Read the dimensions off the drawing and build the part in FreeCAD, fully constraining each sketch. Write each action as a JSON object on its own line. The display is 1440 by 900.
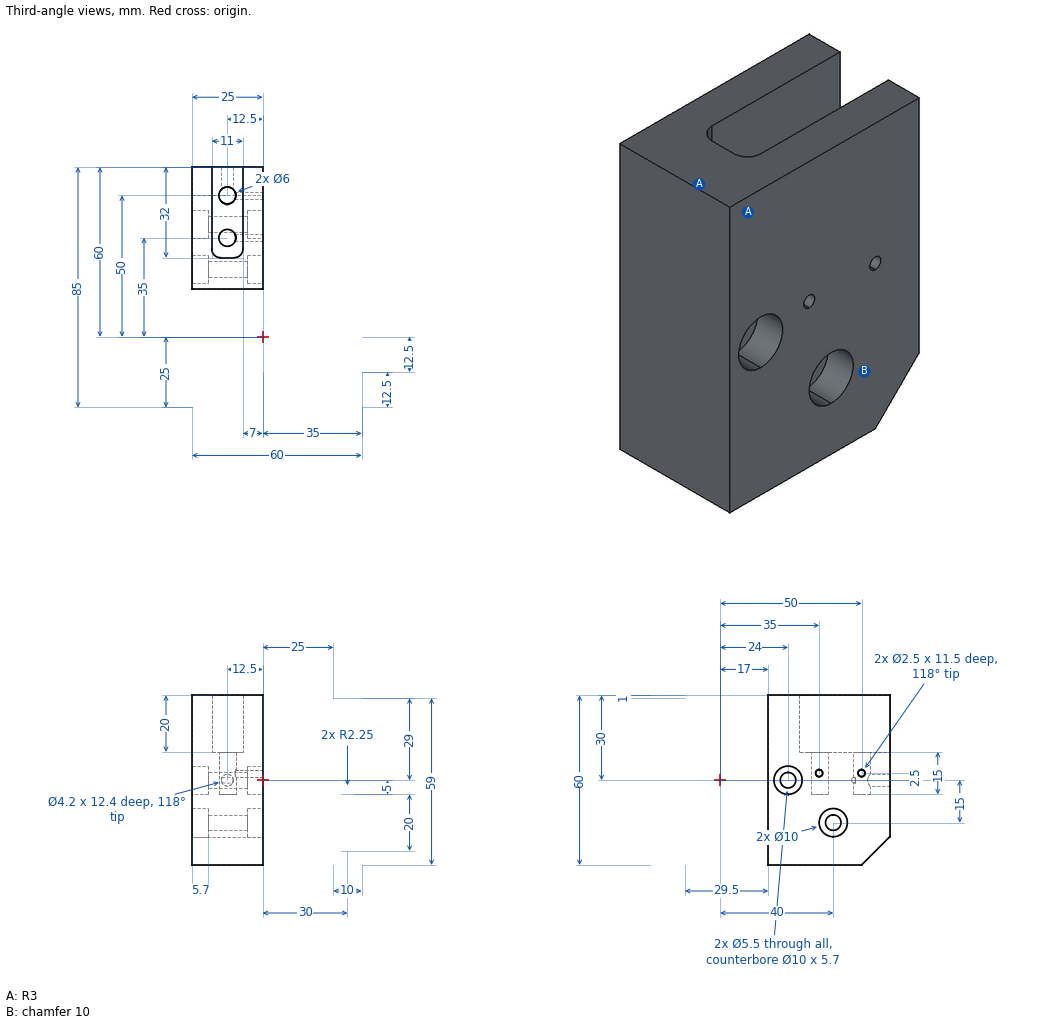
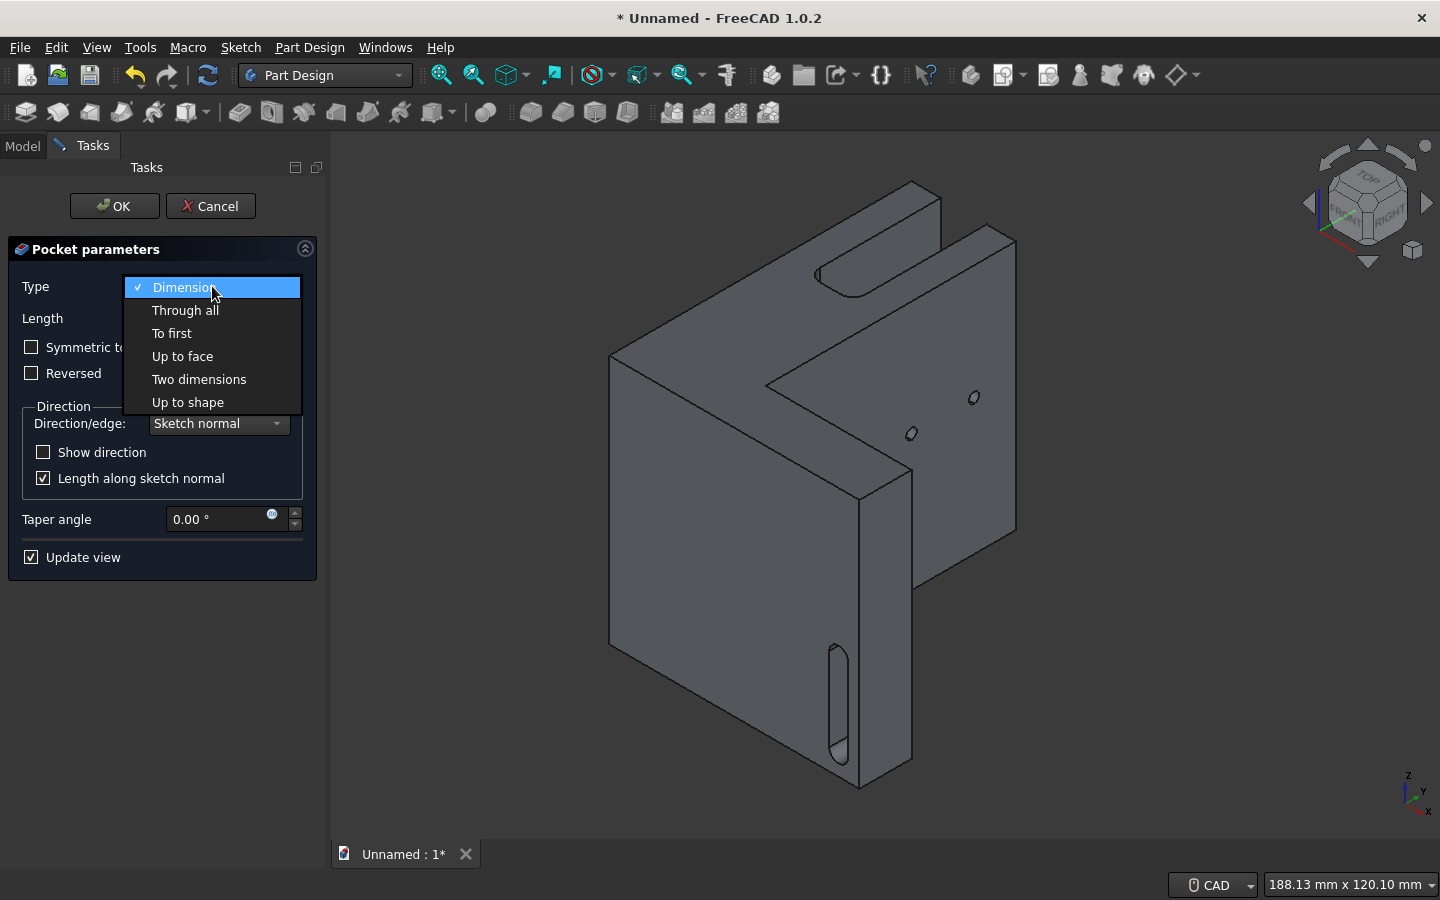
{"action": "left_click", "coordinate": [212, 310]}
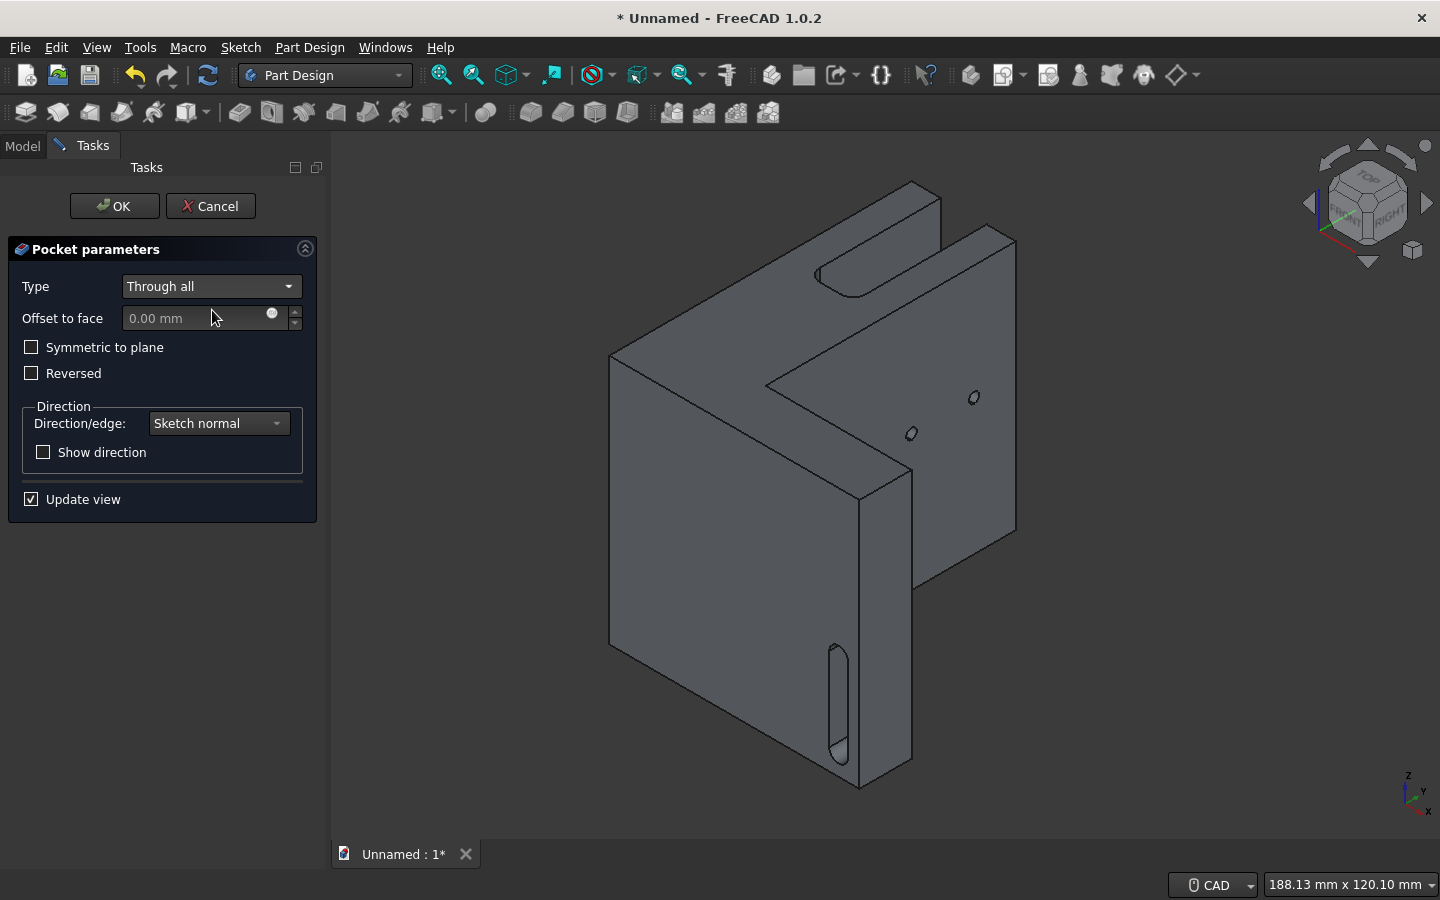
{"action": "left_click", "coordinate": [115, 206]}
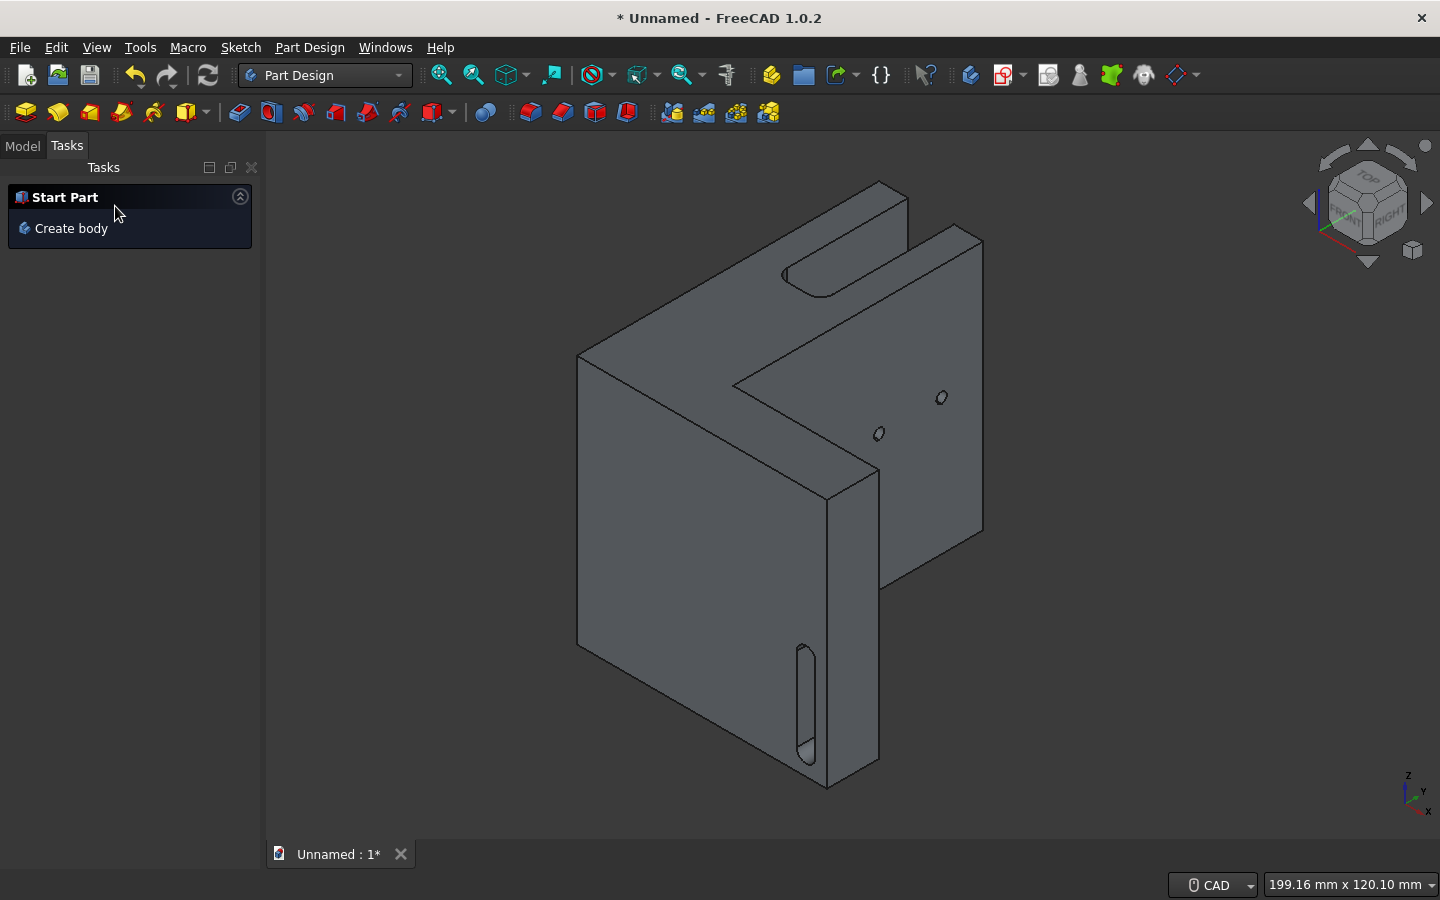
{"action": "left_click", "coordinate": [738, 323]}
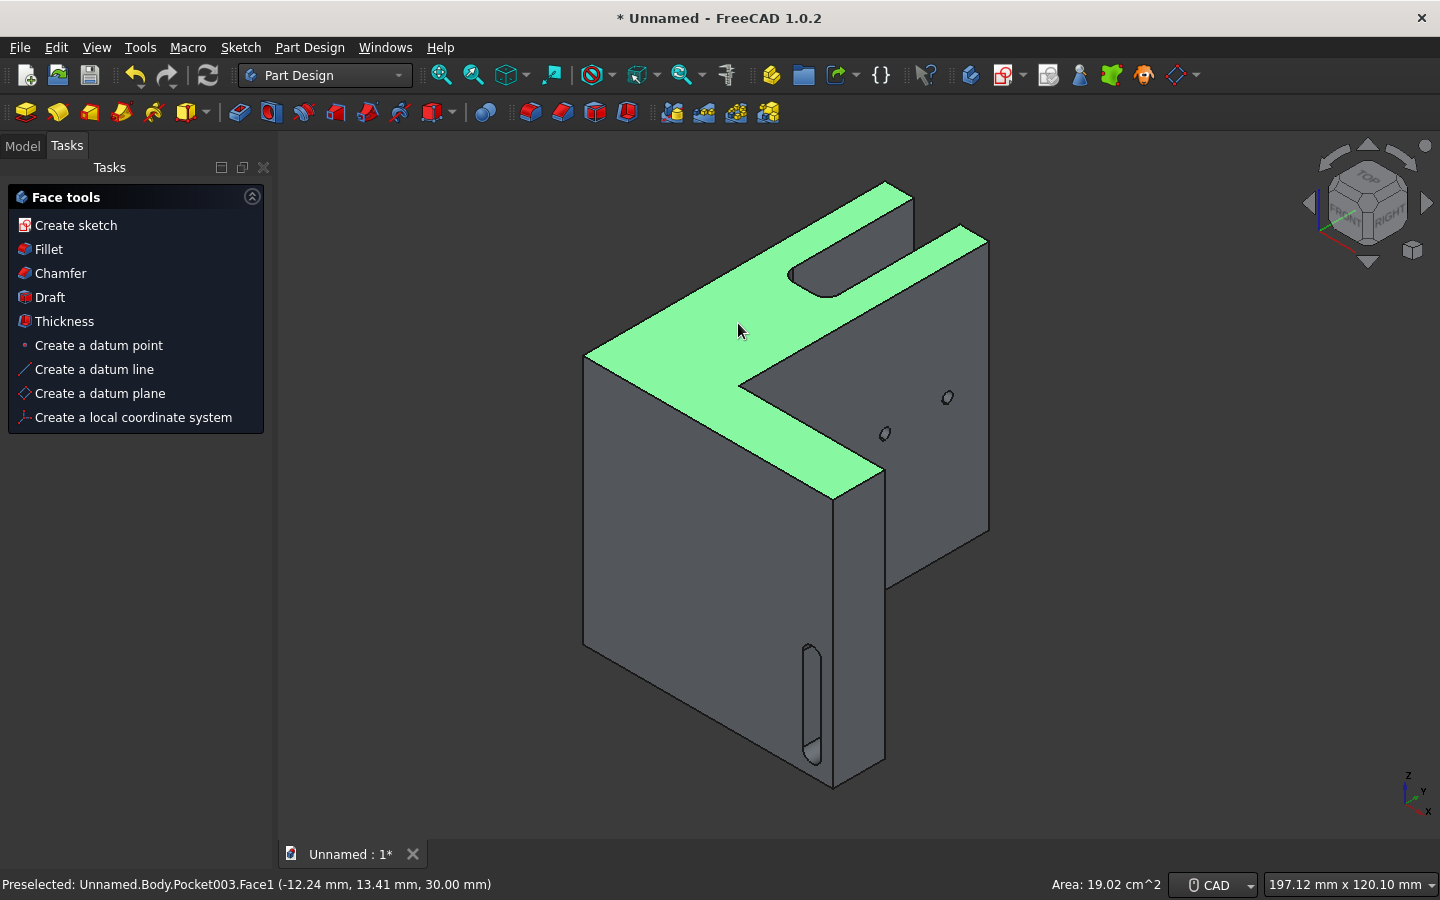
{"action": "left_click", "coordinate": [1004, 76]}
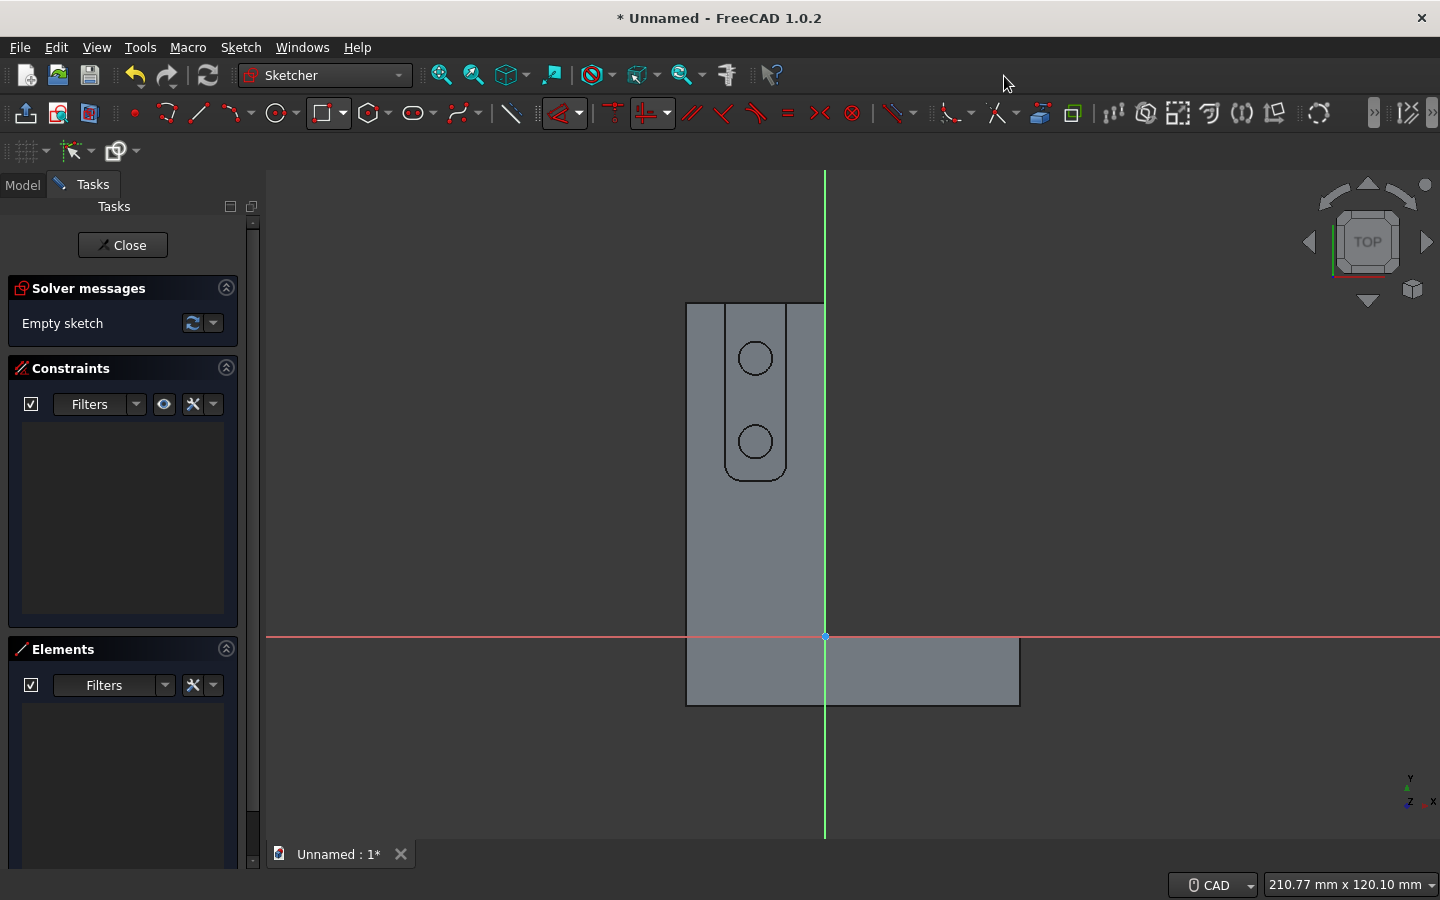
{"action": "scroll", "coordinate": [982, 744], "scroll_direction": "up", "scroll_amount": 6}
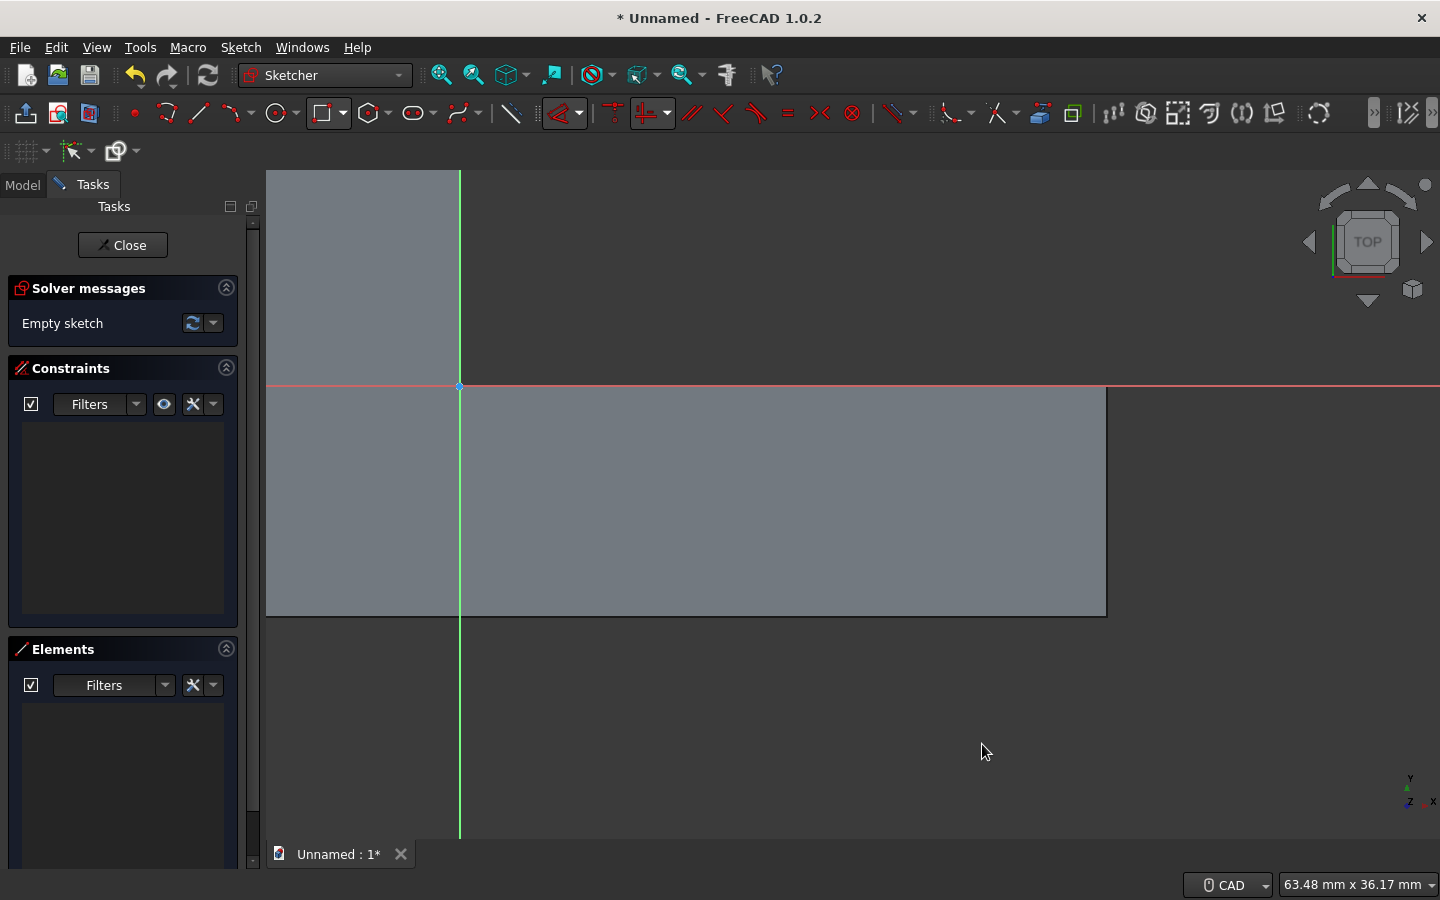
{"action": "left_click", "coordinate": [322, 114]}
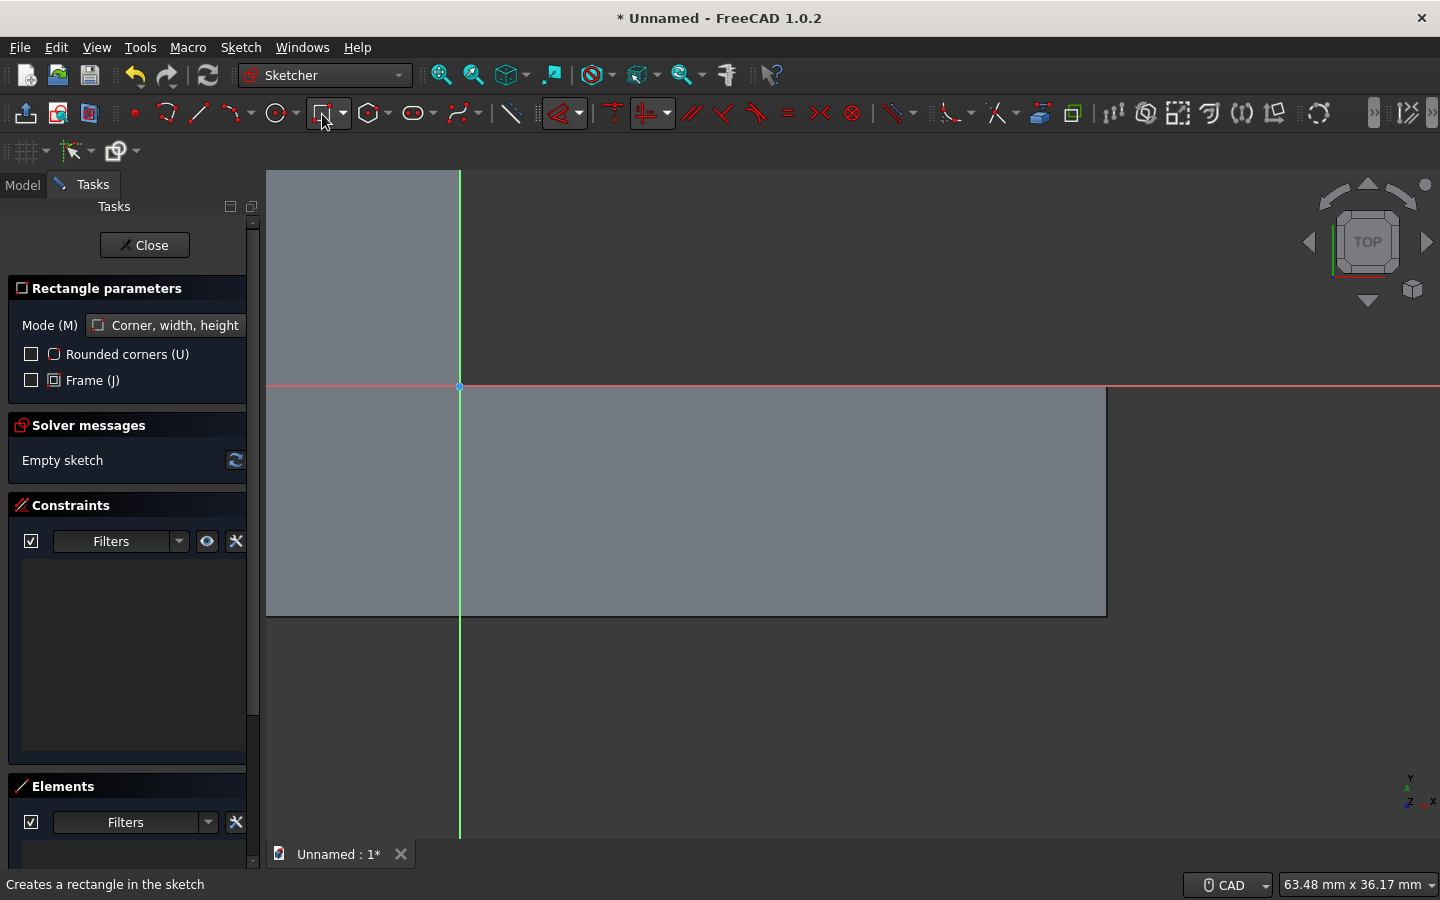
{"action": "left_click", "coordinate": [460, 386]}
{"action": "mouse_move", "coordinate": [1107, 617]}